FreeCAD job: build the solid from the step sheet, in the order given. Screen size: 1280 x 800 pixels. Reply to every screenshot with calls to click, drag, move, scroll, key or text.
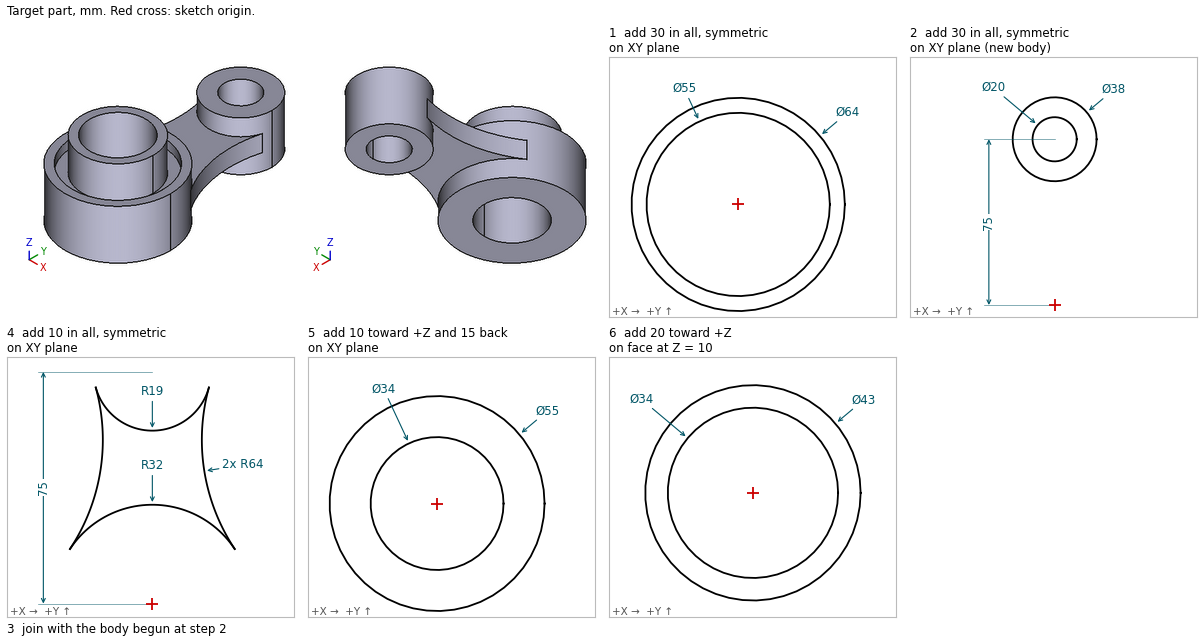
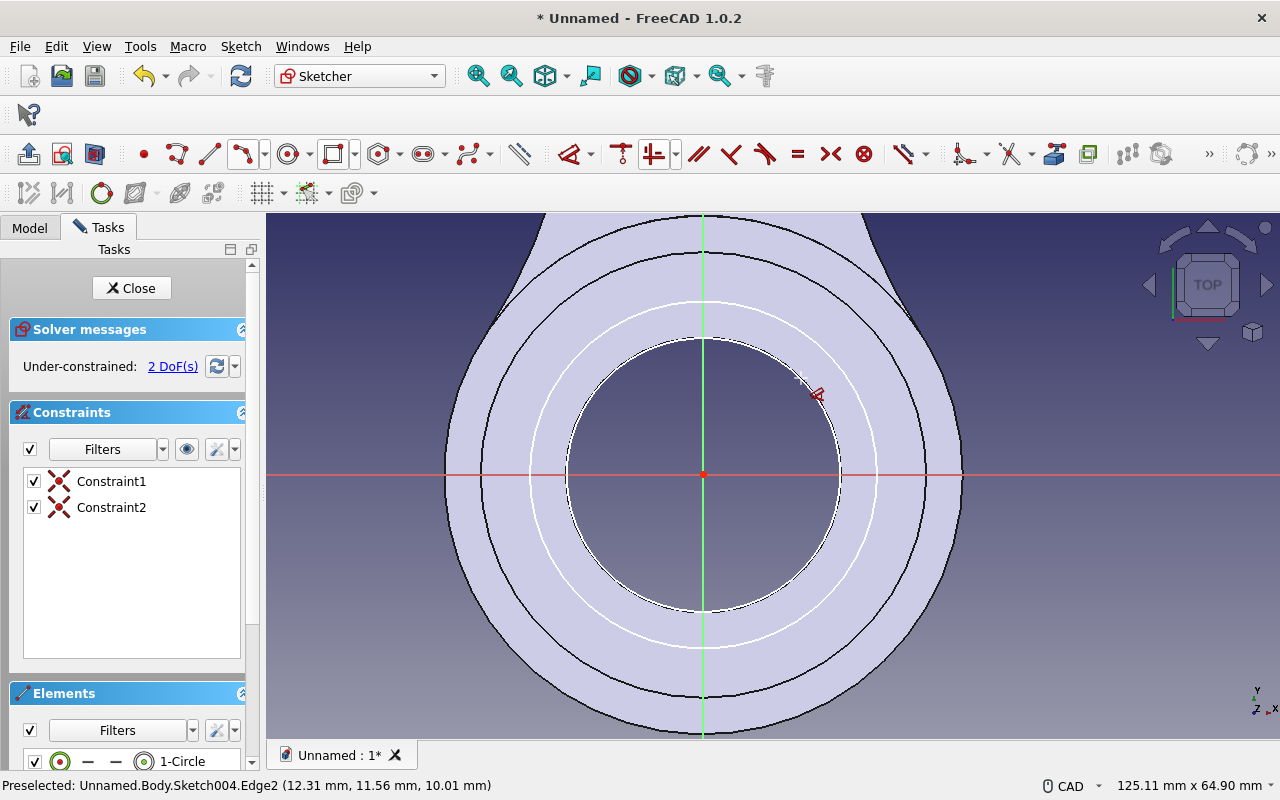
click(826, 352)
click(849, 329)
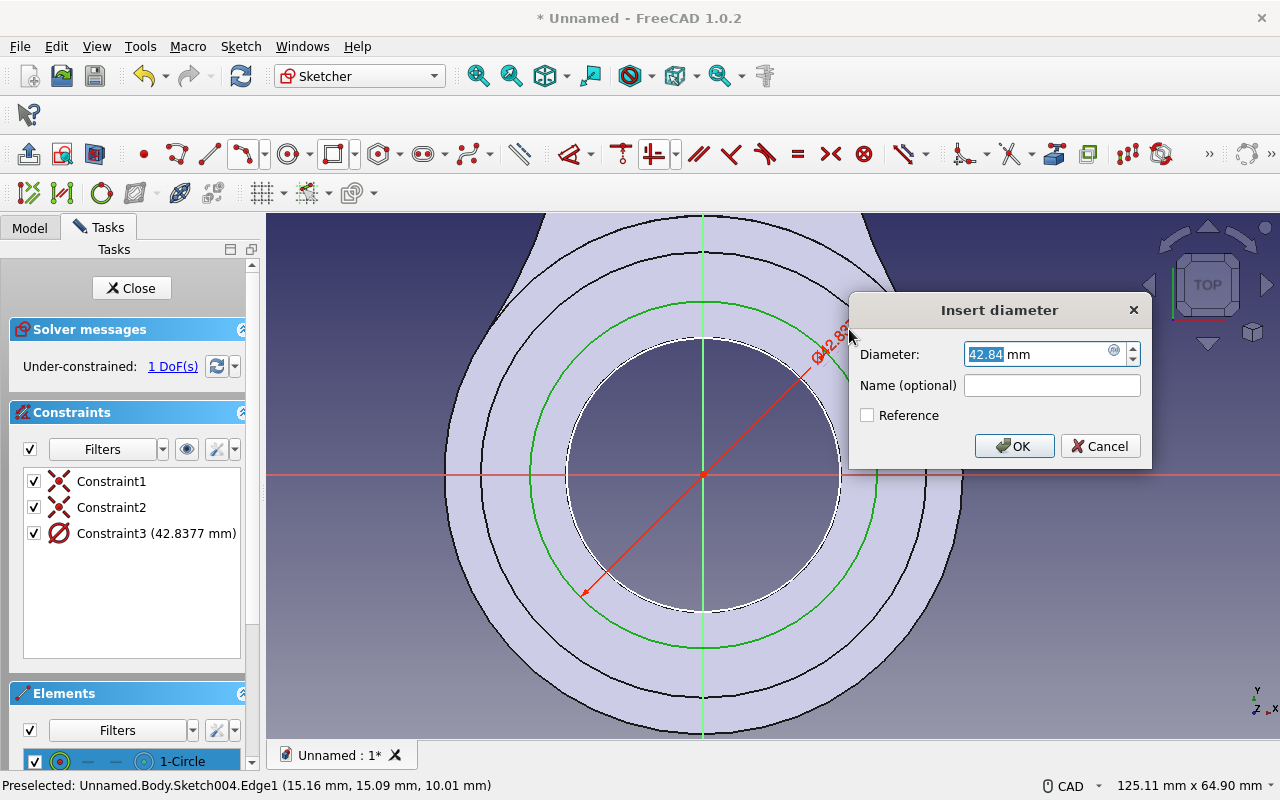
text(43)
key(Return)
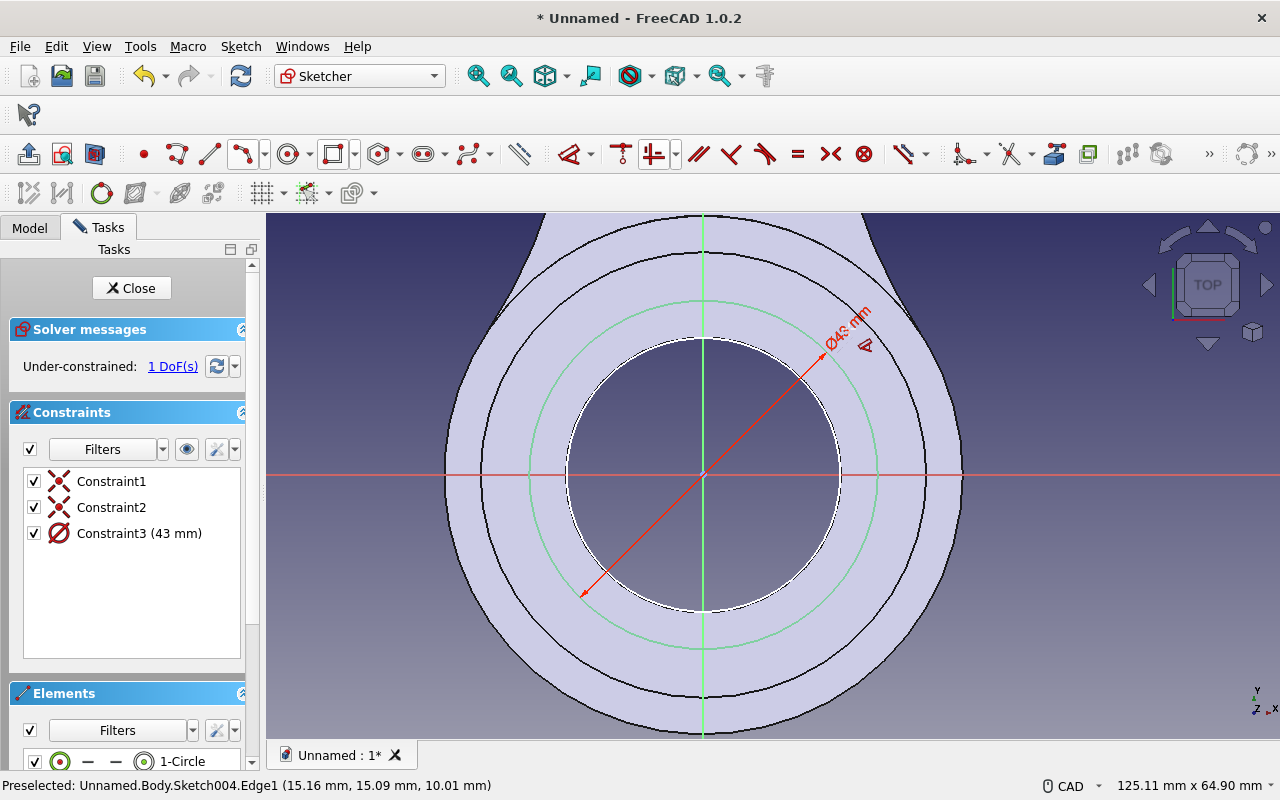
click(800, 378)
click(887, 421)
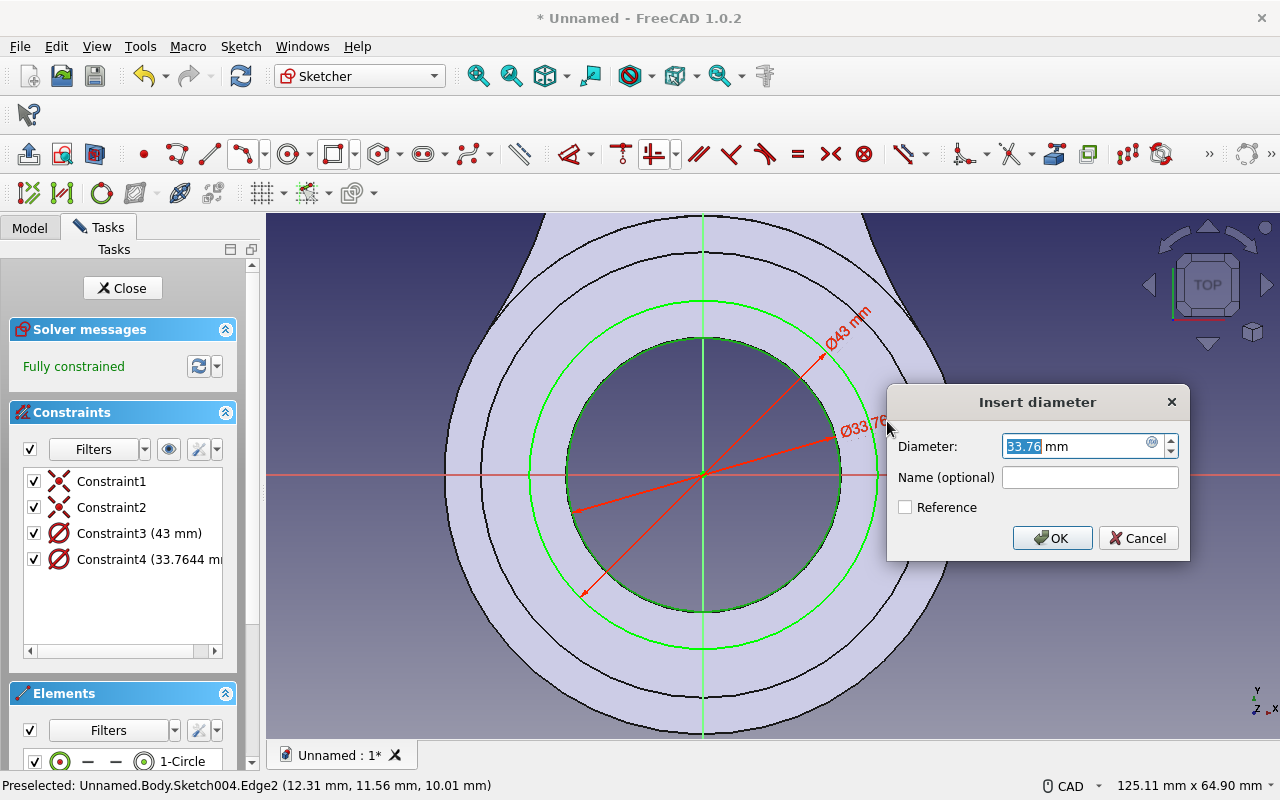
text(34)
key(Return)
key(Escape)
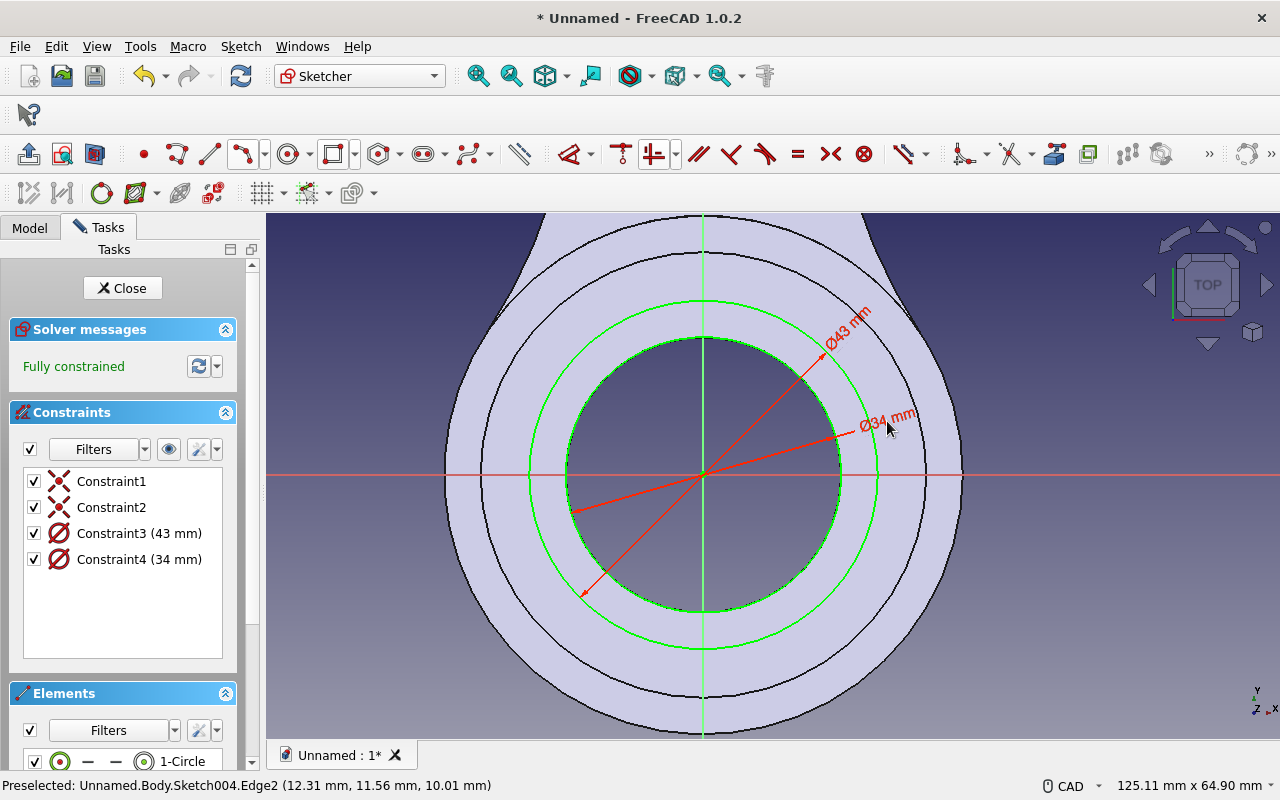
click(123, 288)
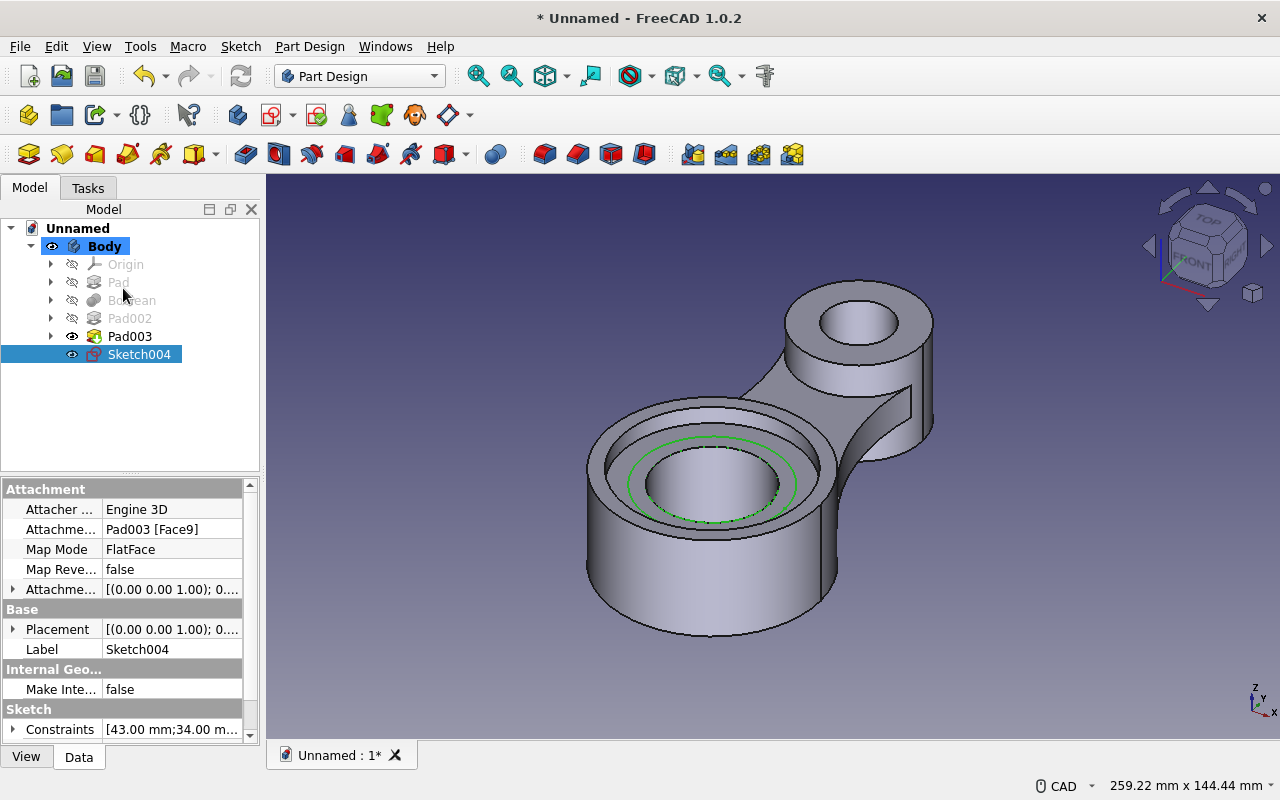
click(29, 154)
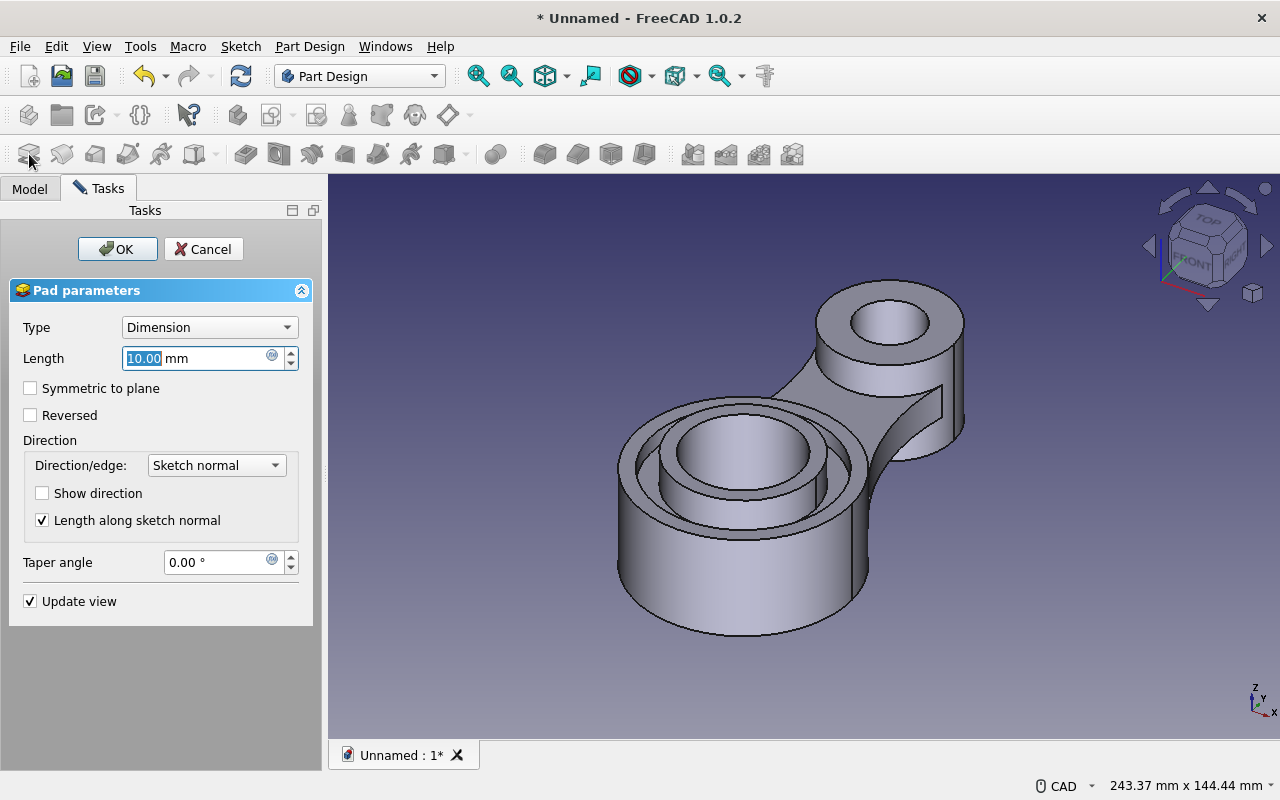
text(20)
key(Tab)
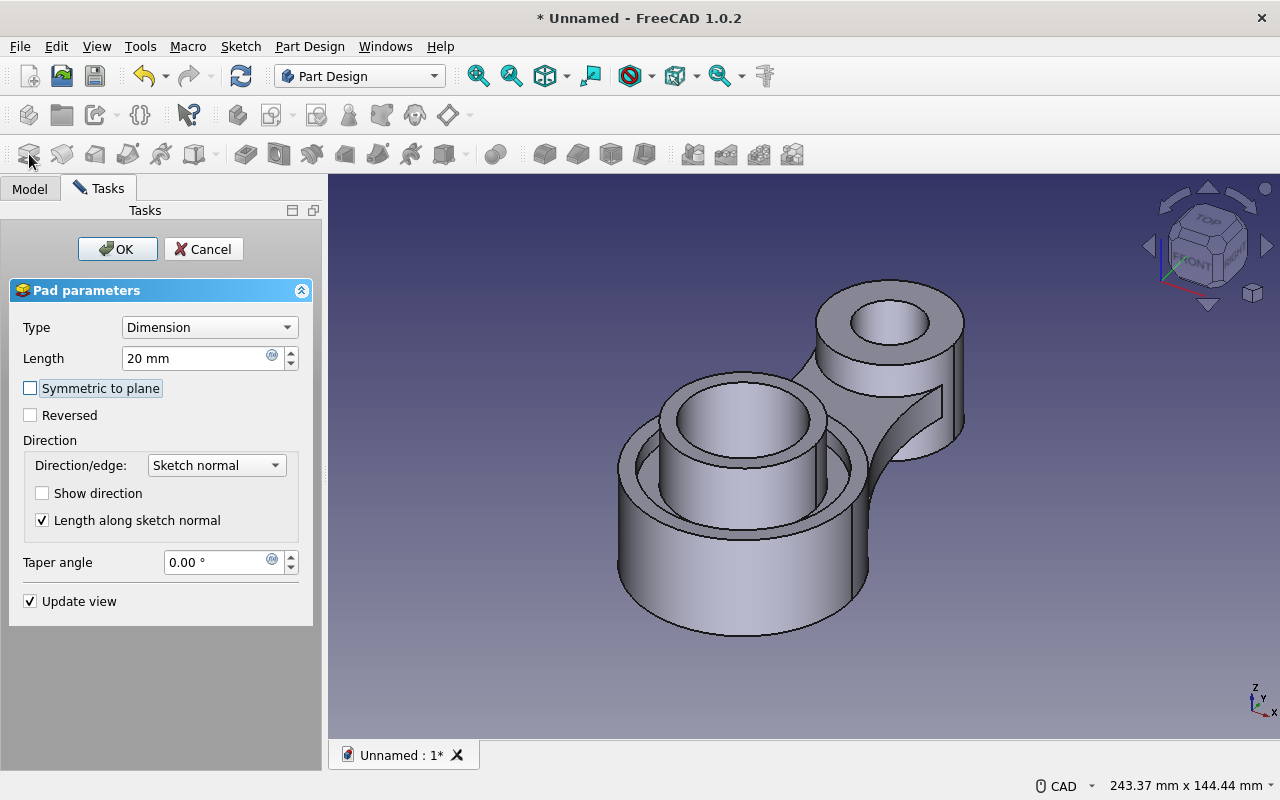
click(118, 249)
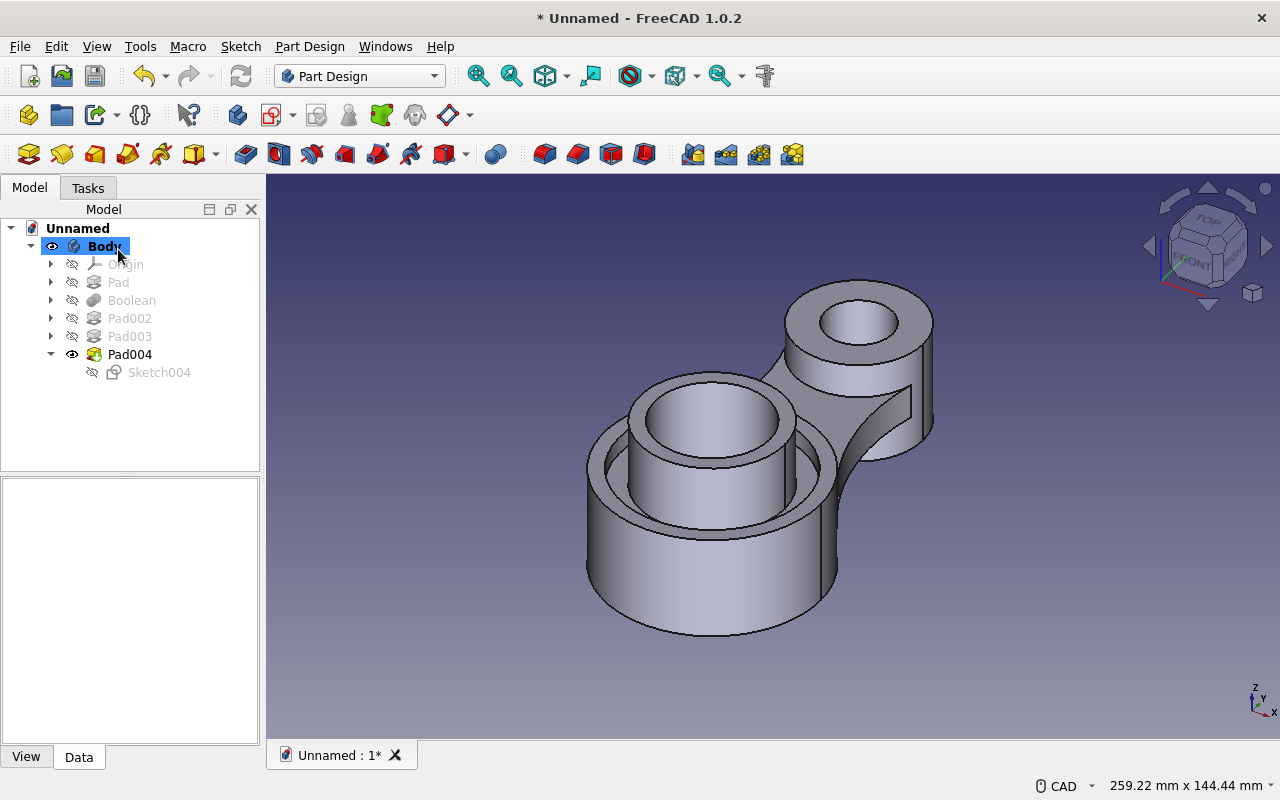
key(0)